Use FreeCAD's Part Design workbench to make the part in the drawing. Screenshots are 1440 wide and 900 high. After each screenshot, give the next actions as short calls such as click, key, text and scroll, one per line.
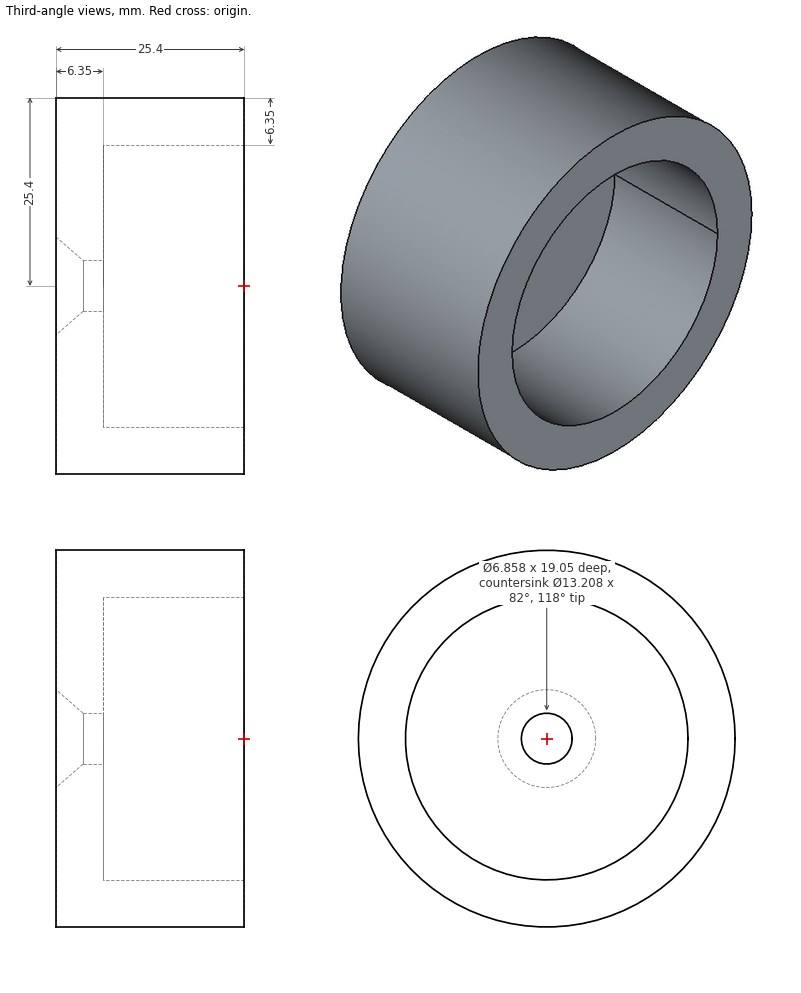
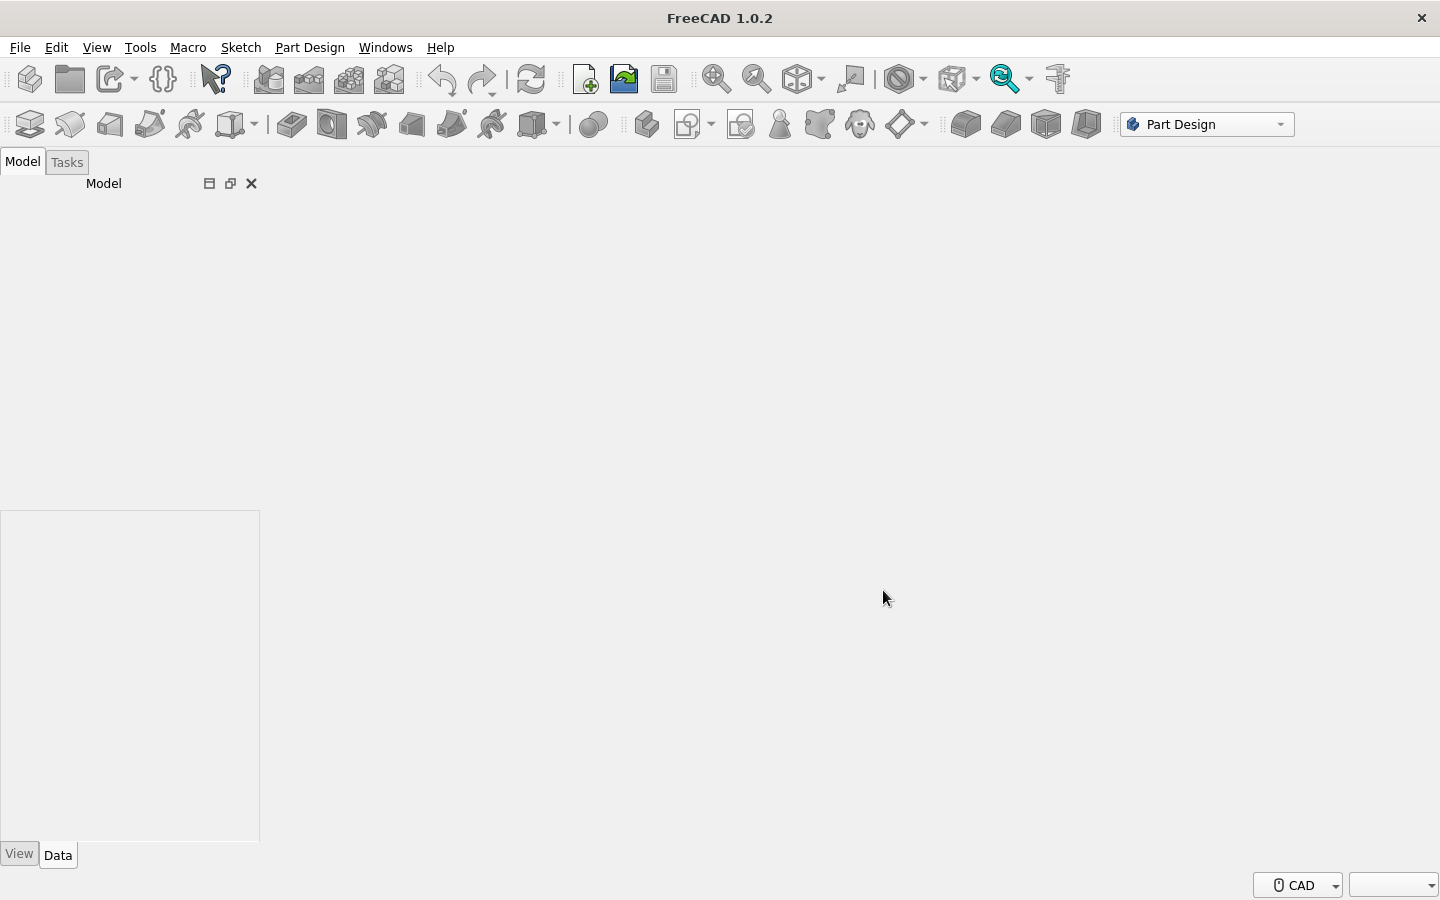
key(ctrl+n)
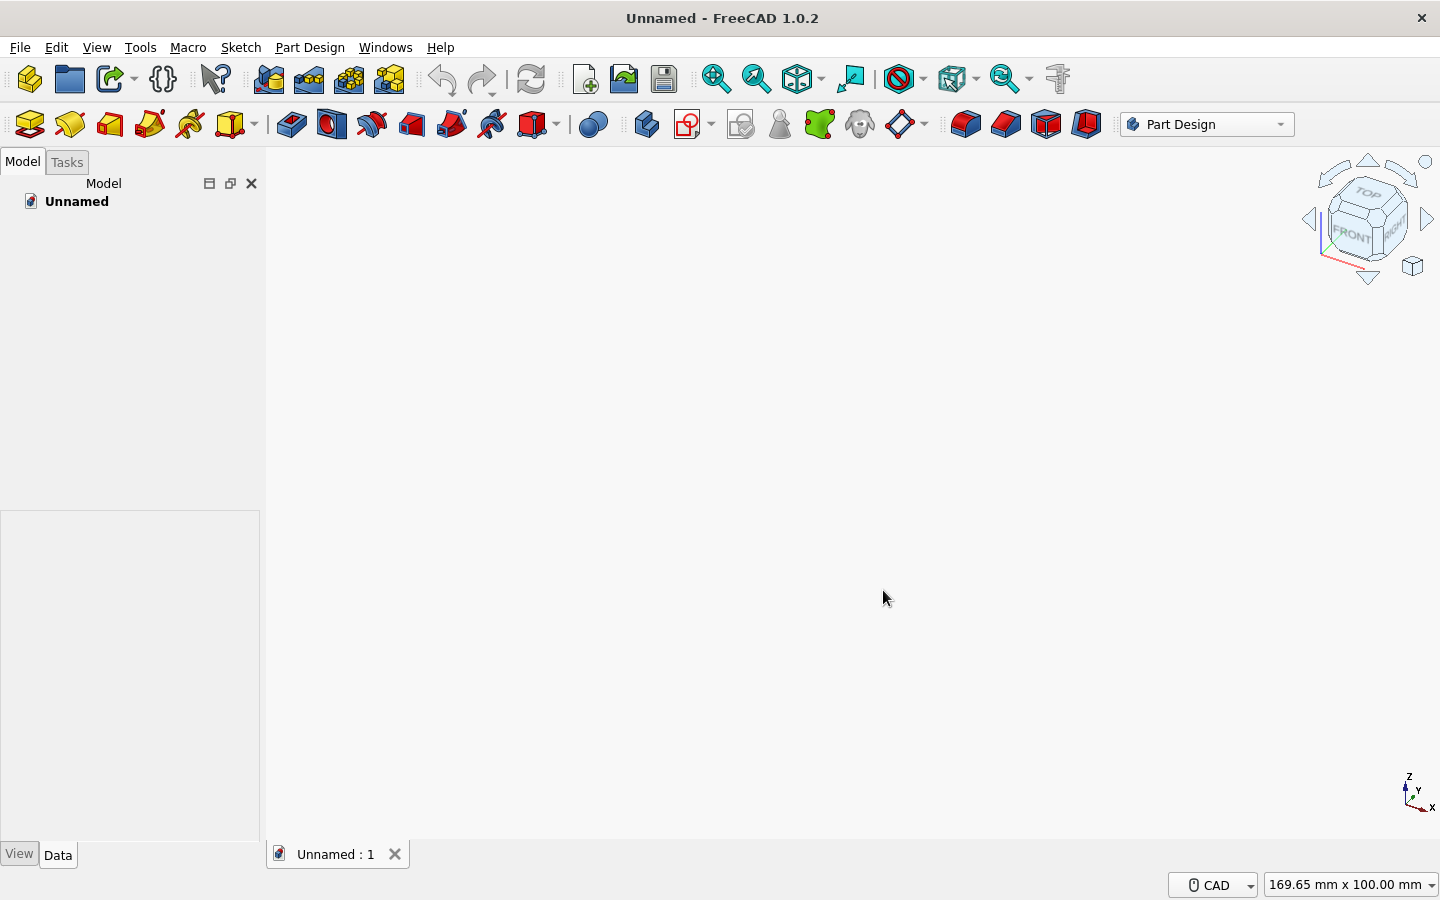
click(688, 124)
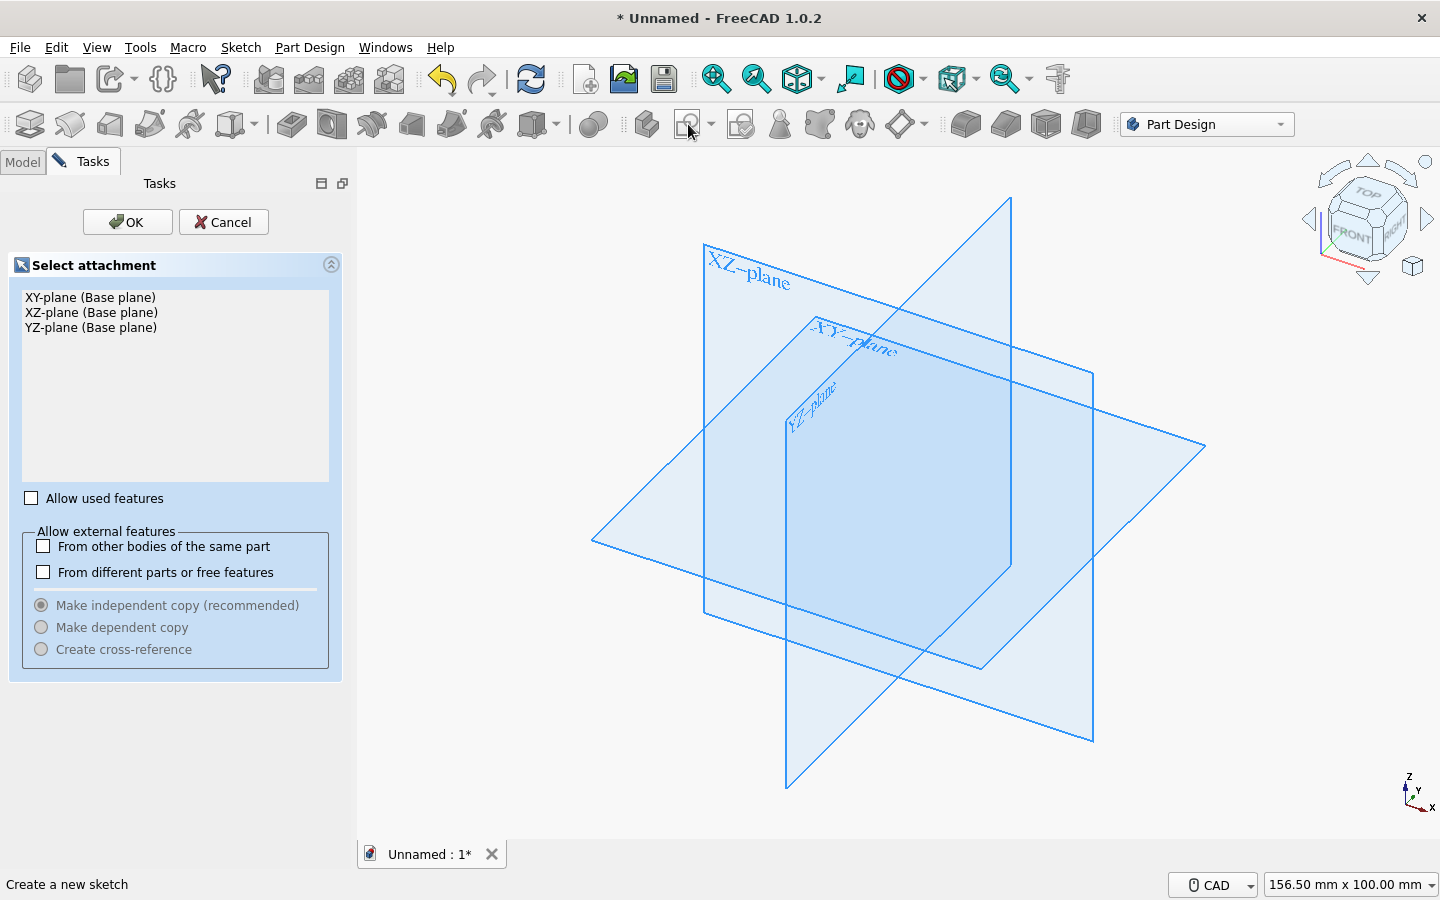
click(82, 298)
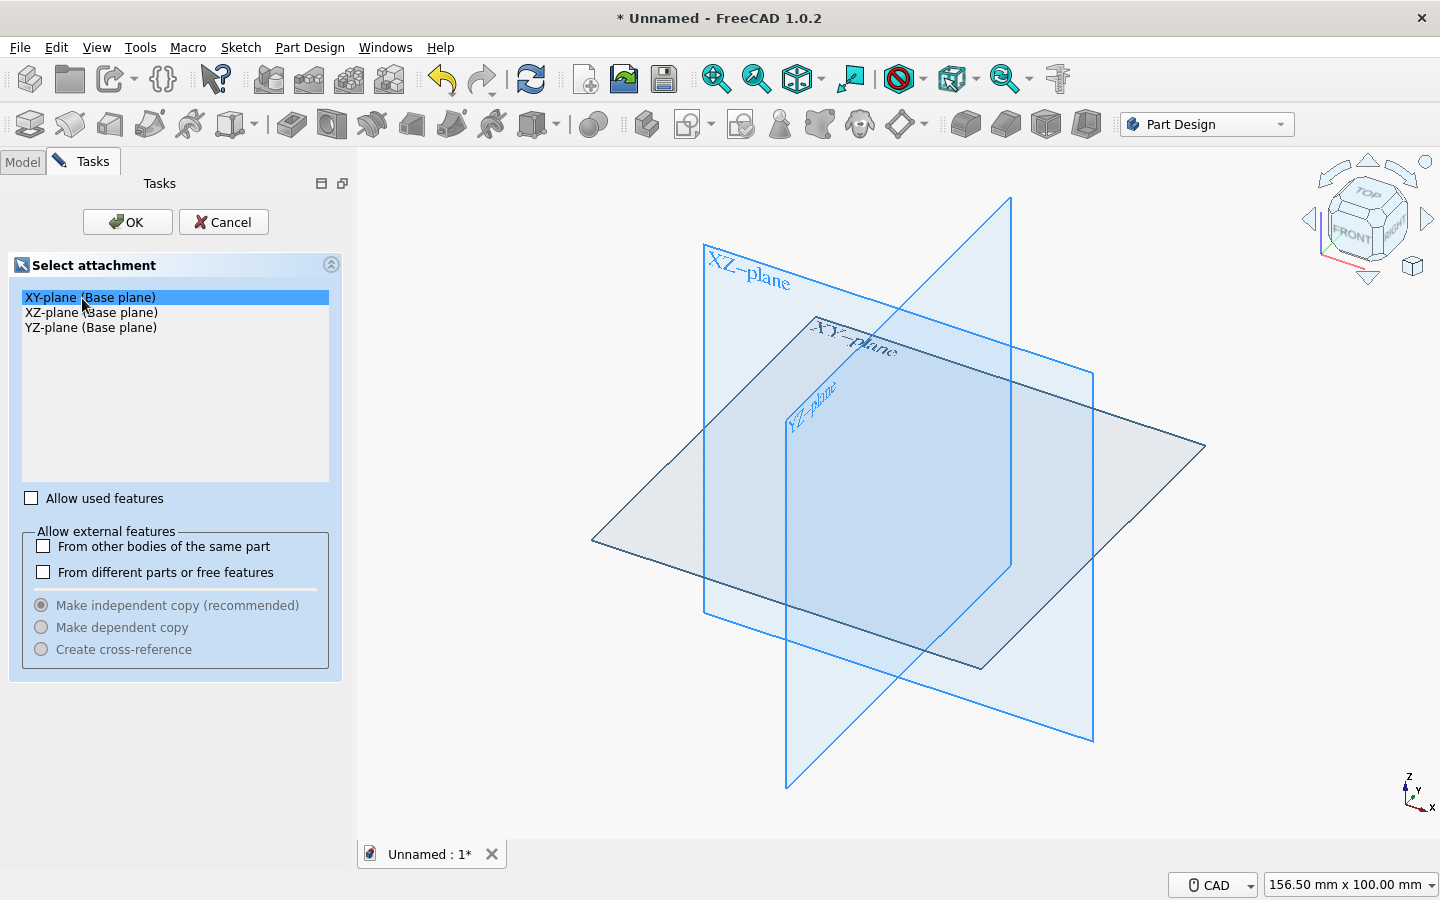
click(128, 222)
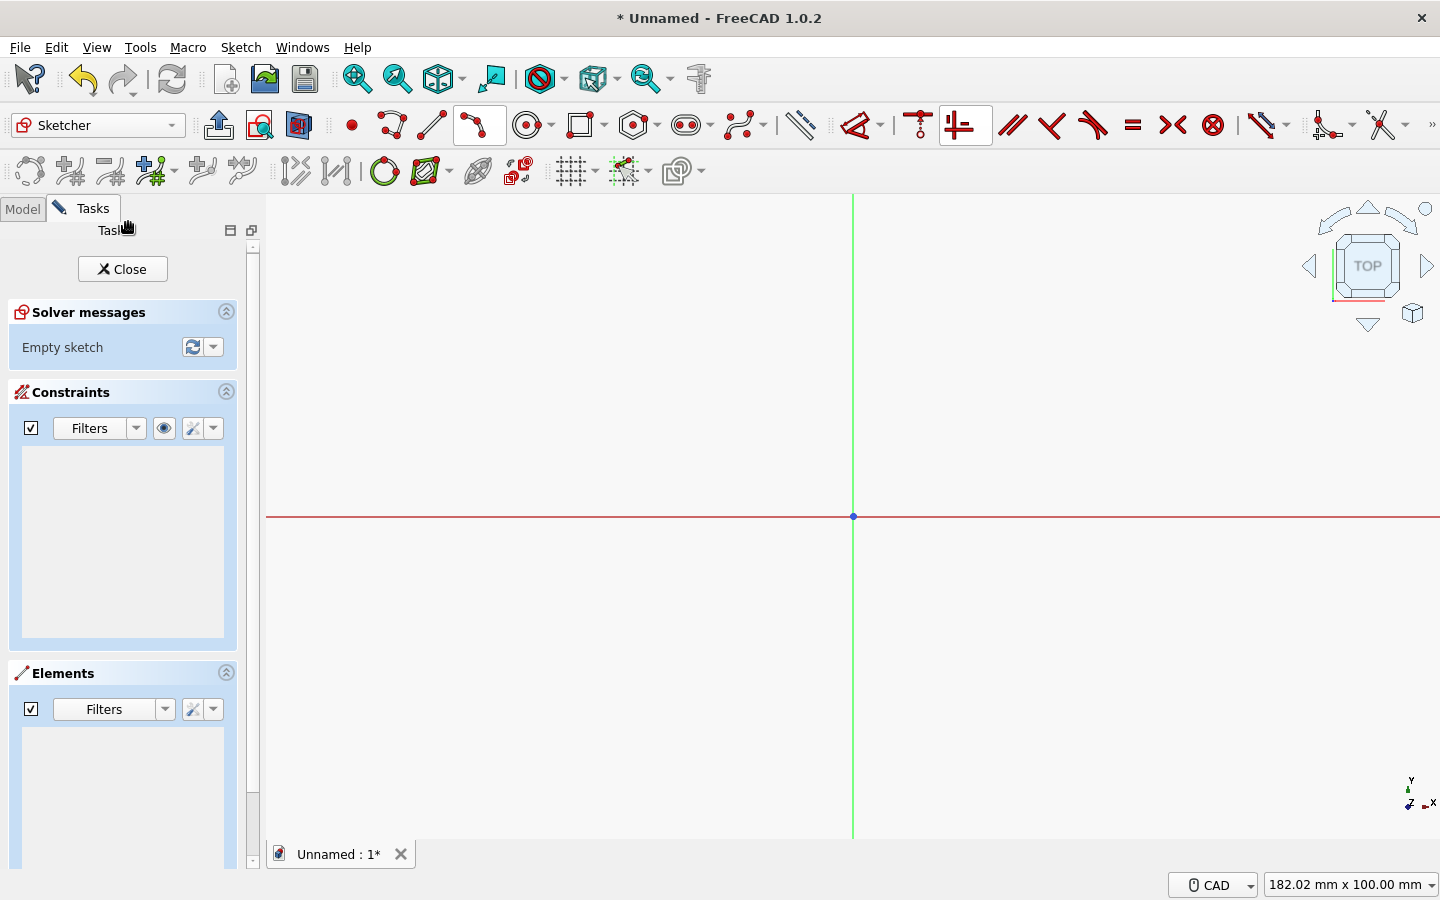
scroll(763, 387, up, 5)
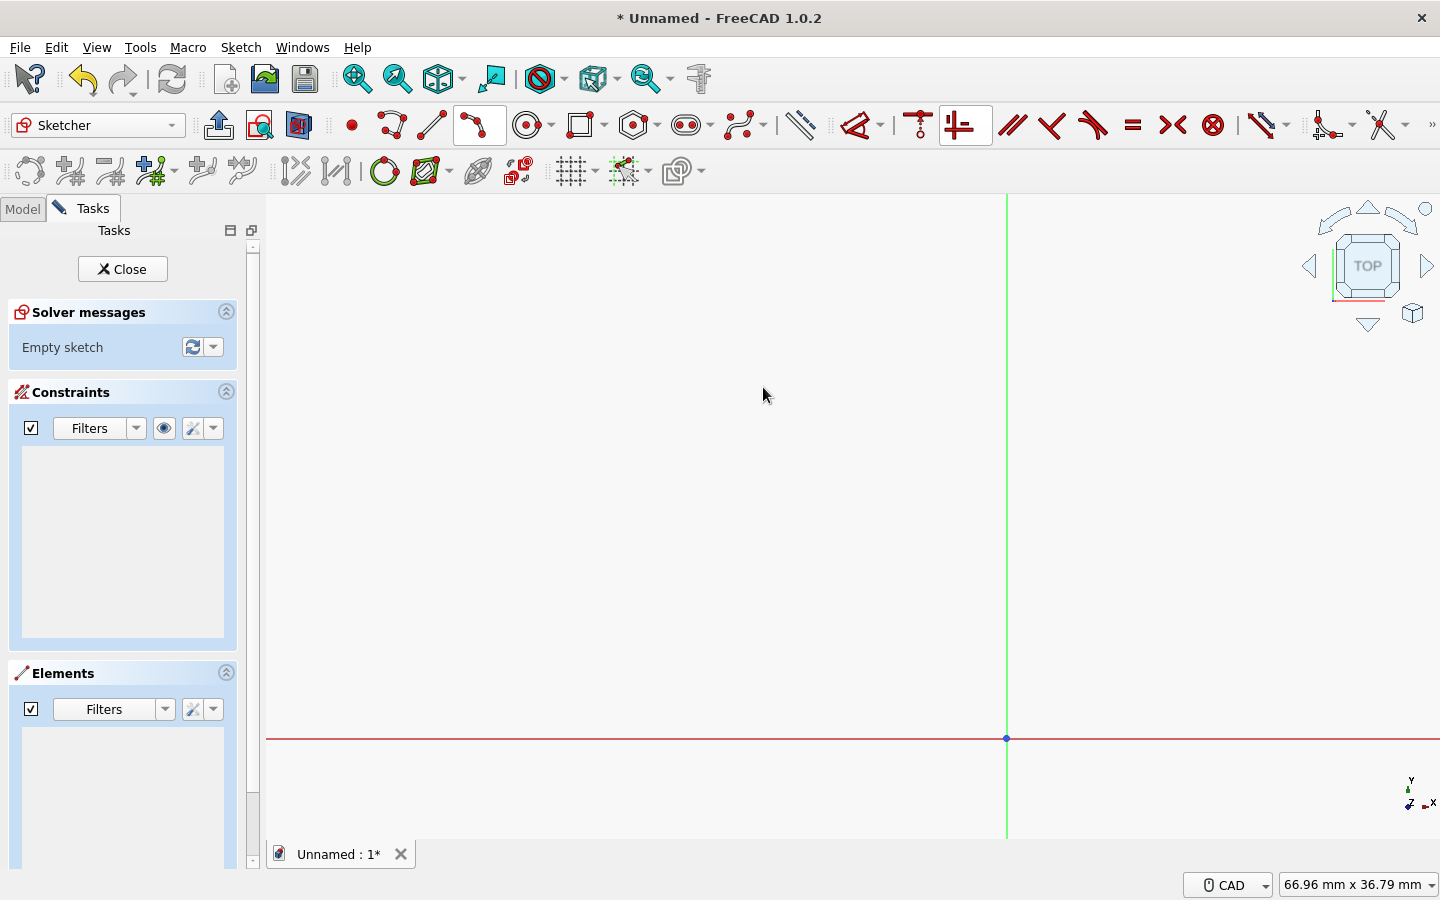
click(392, 126)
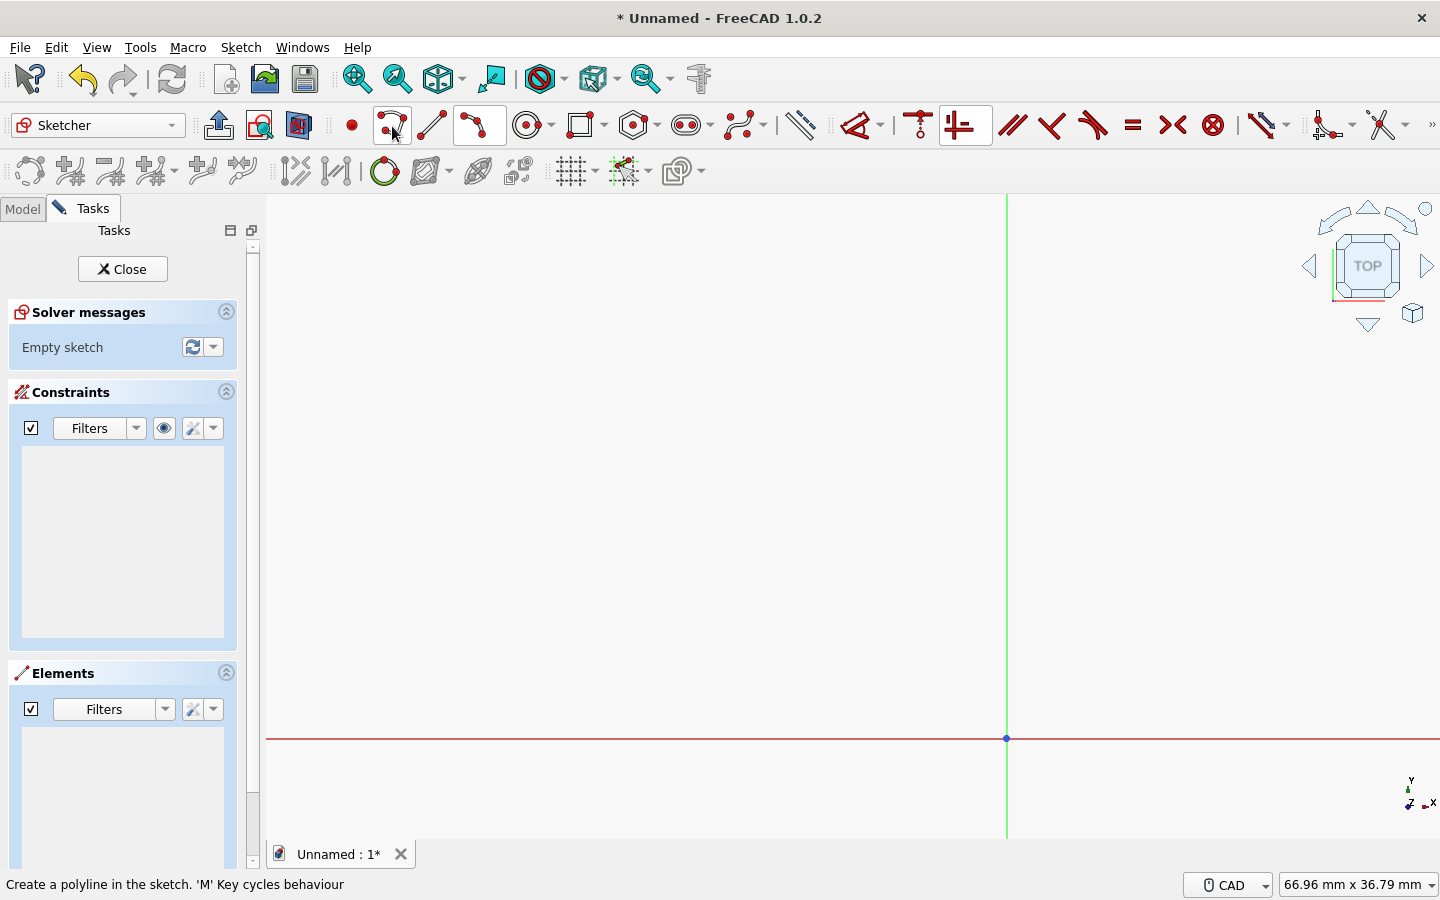
click(673, 739)
click(673, 405)
click(1007, 405)
click(998, 293)
click(562, 293)
click(562, 730)
click(673, 739)
key(Escape)
key(Escape)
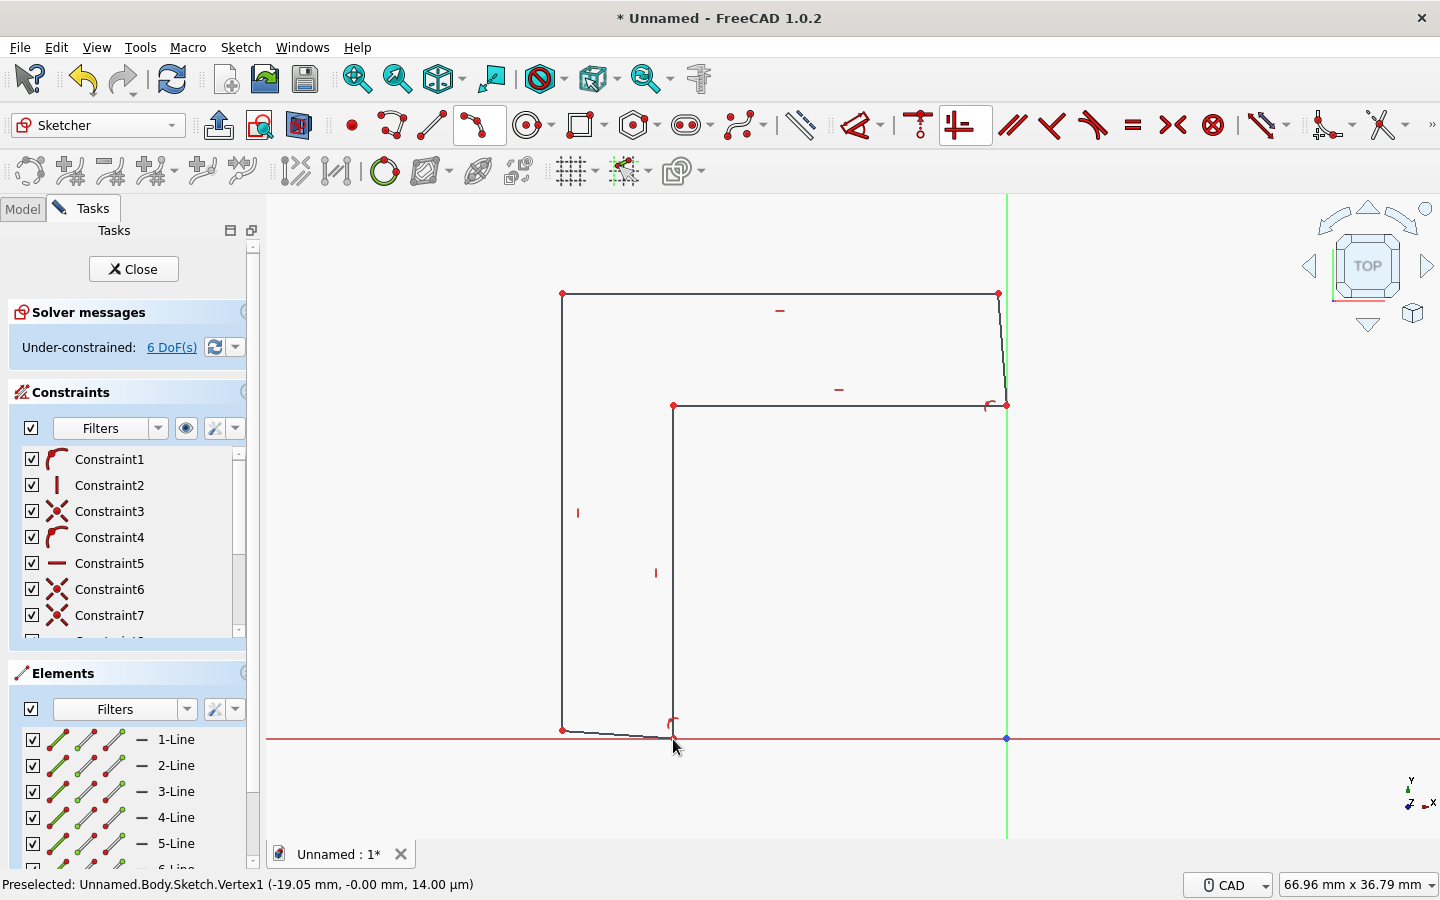
click(1004, 372)